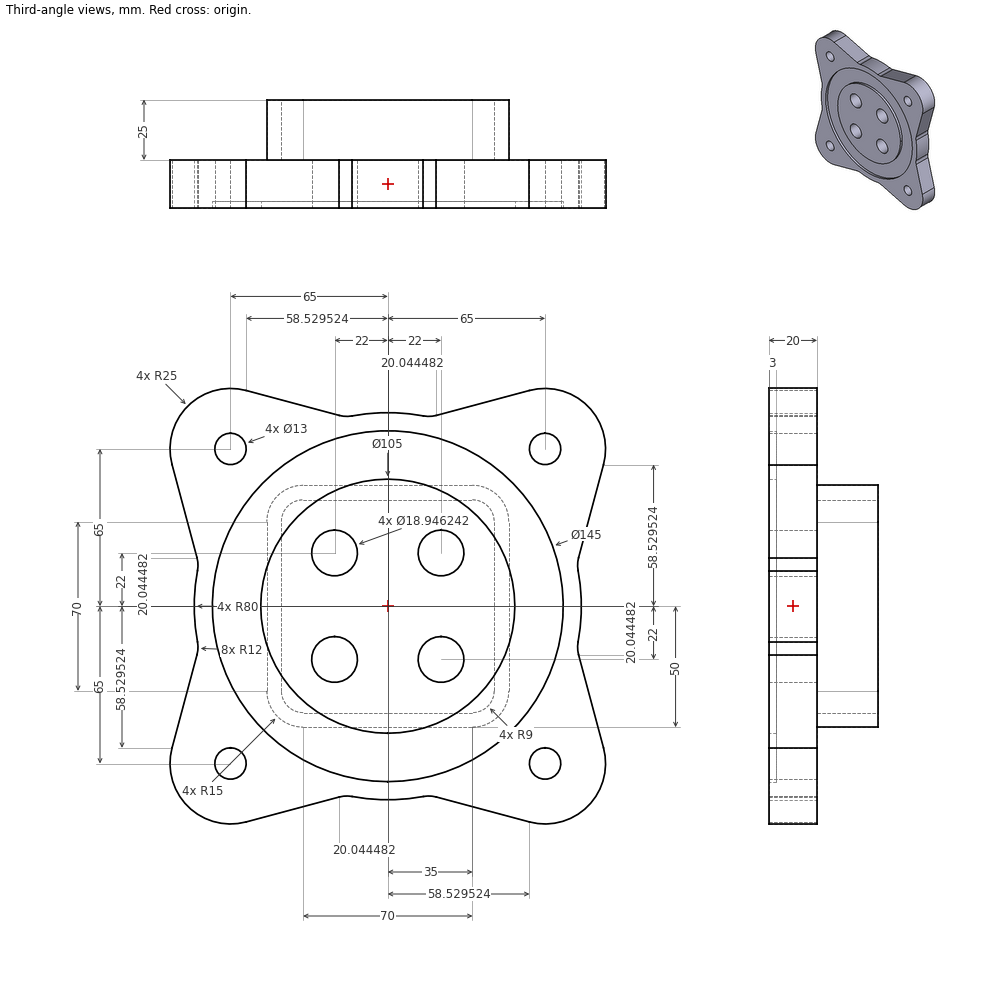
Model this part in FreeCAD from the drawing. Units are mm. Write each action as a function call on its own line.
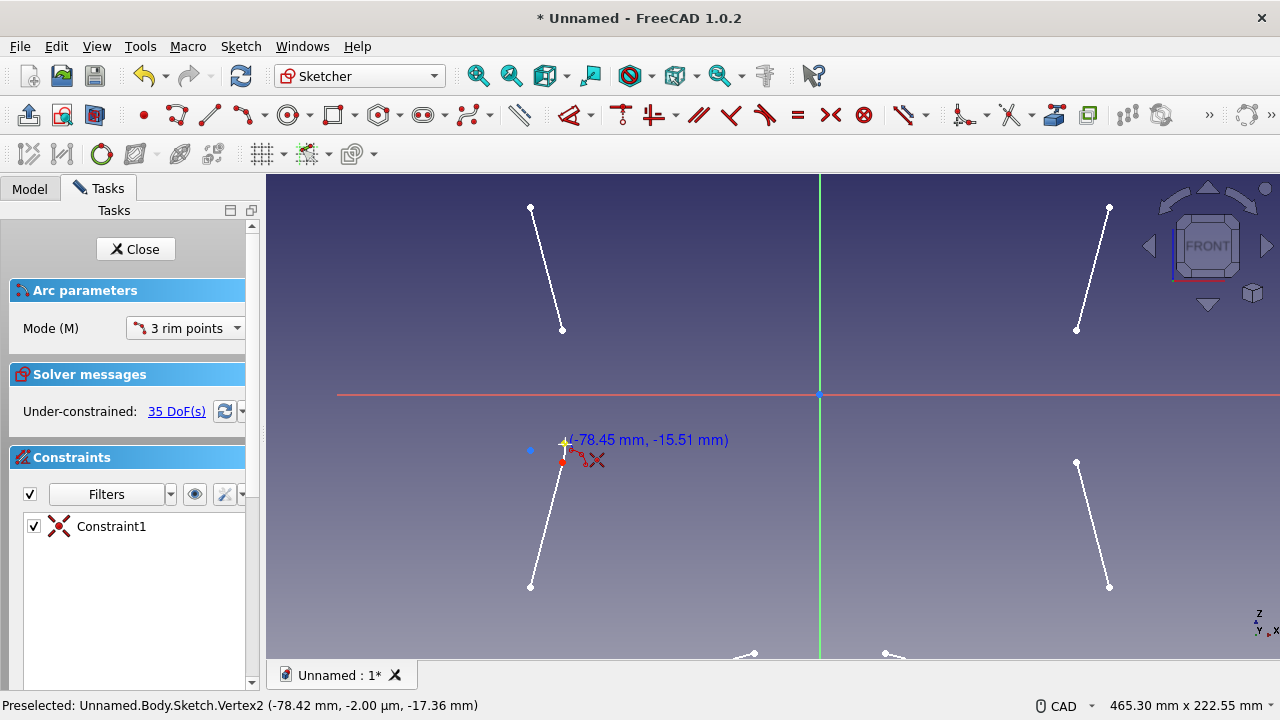
click(564, 444)
click(564, 347)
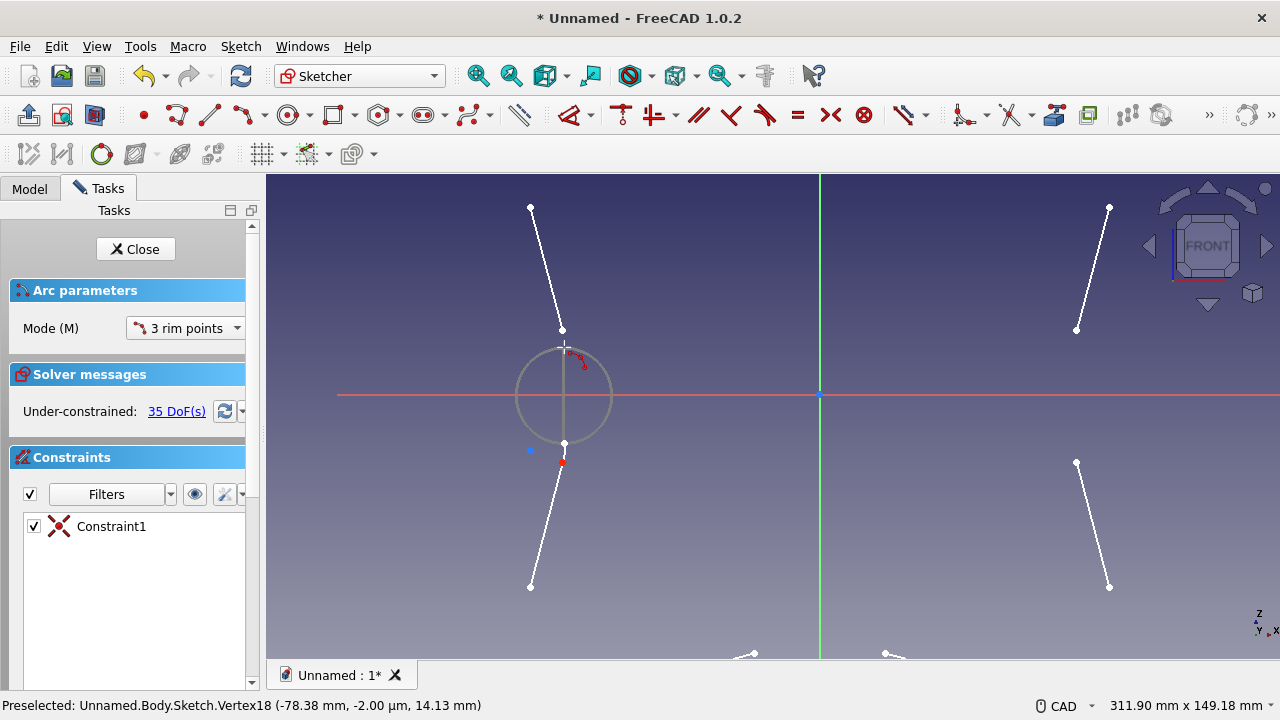
scroll(560, 385, up, 7)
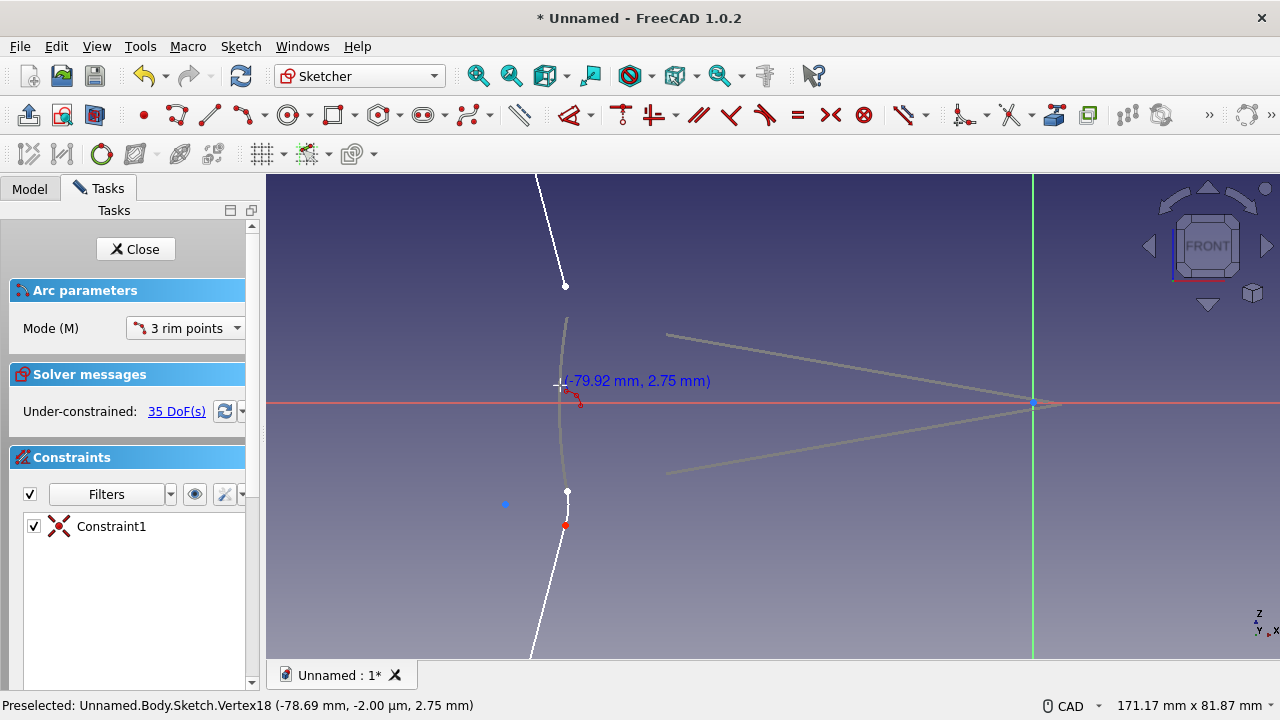
click(559, 385)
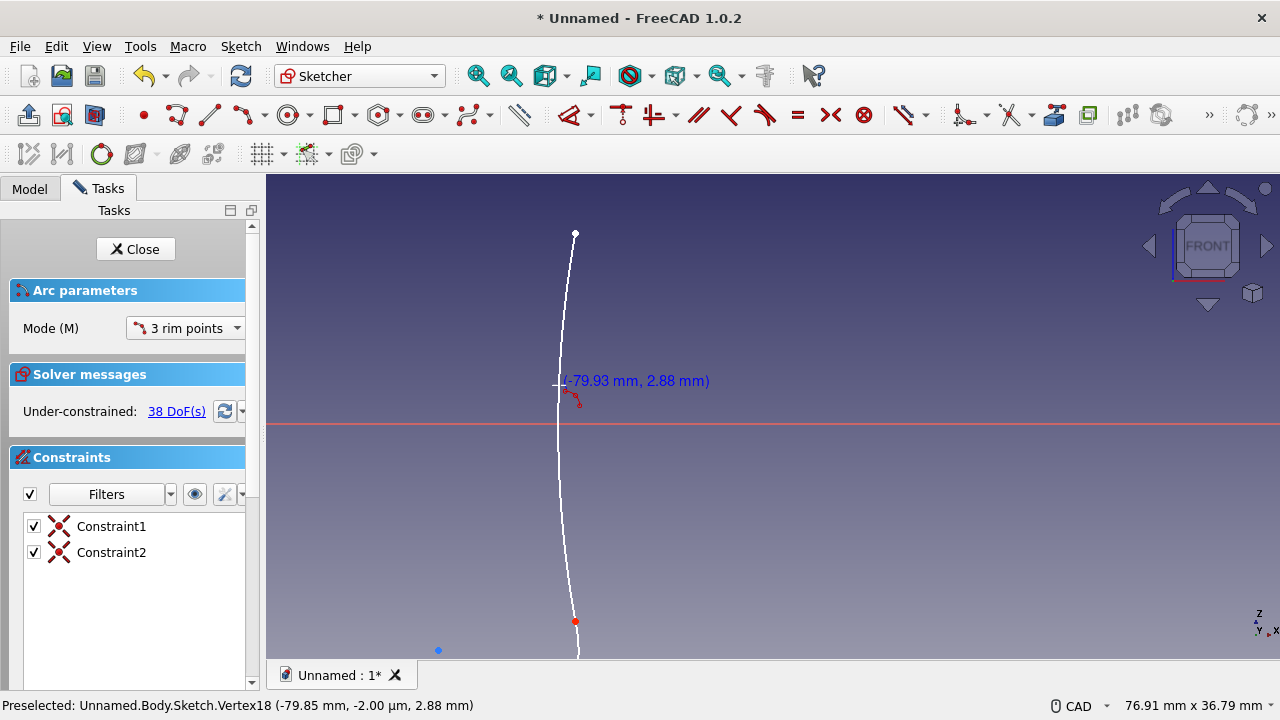
scroll(562, 415, down, 10)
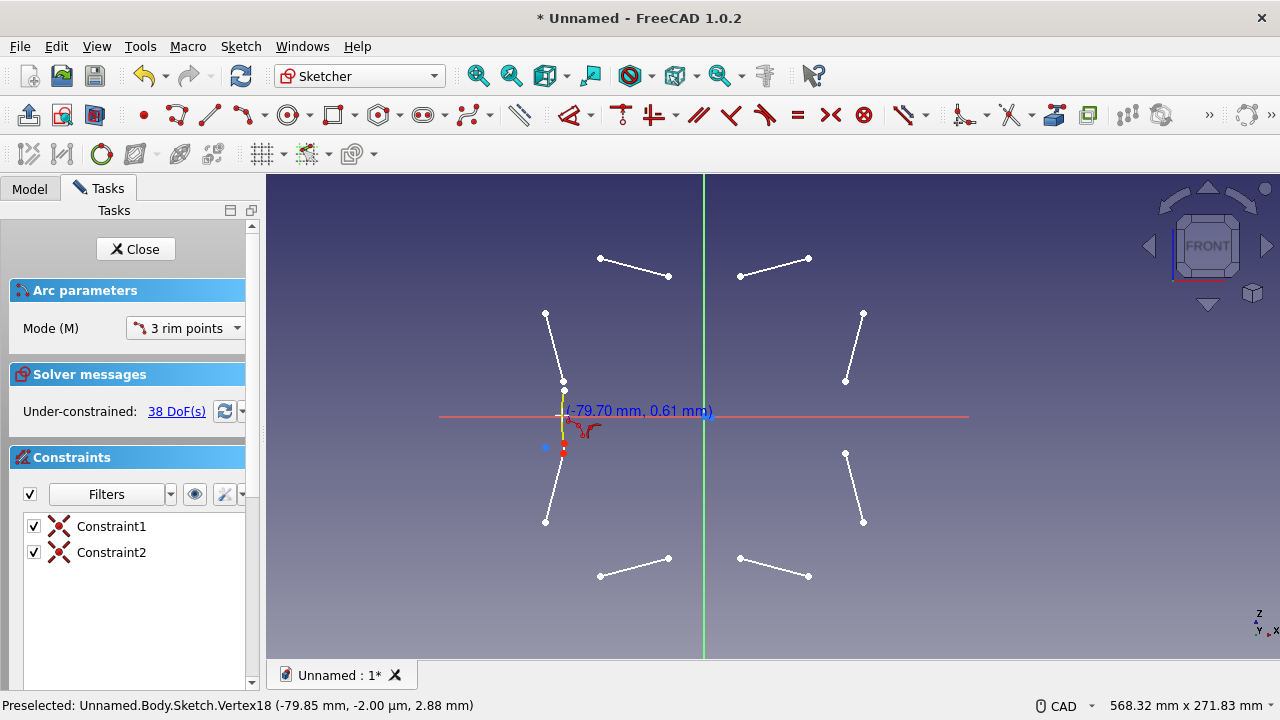
scroll(564, 390, up, 3)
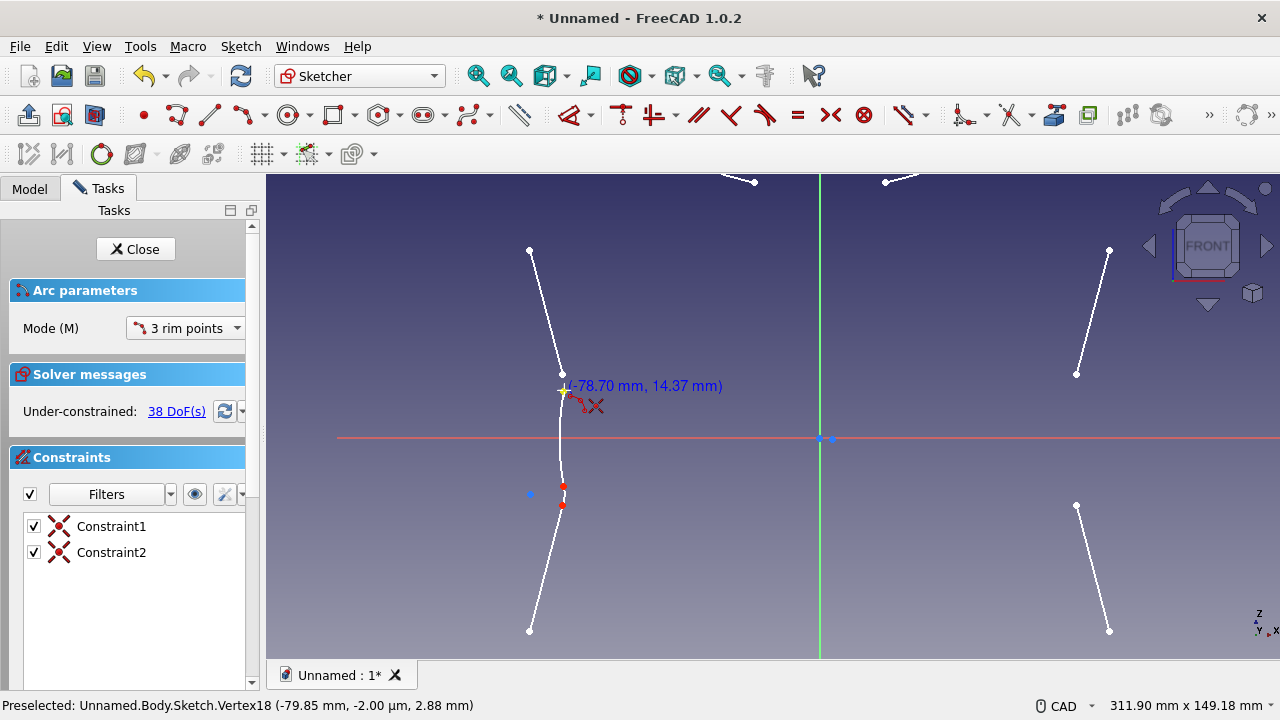
click(564, 391)
click(563, 374)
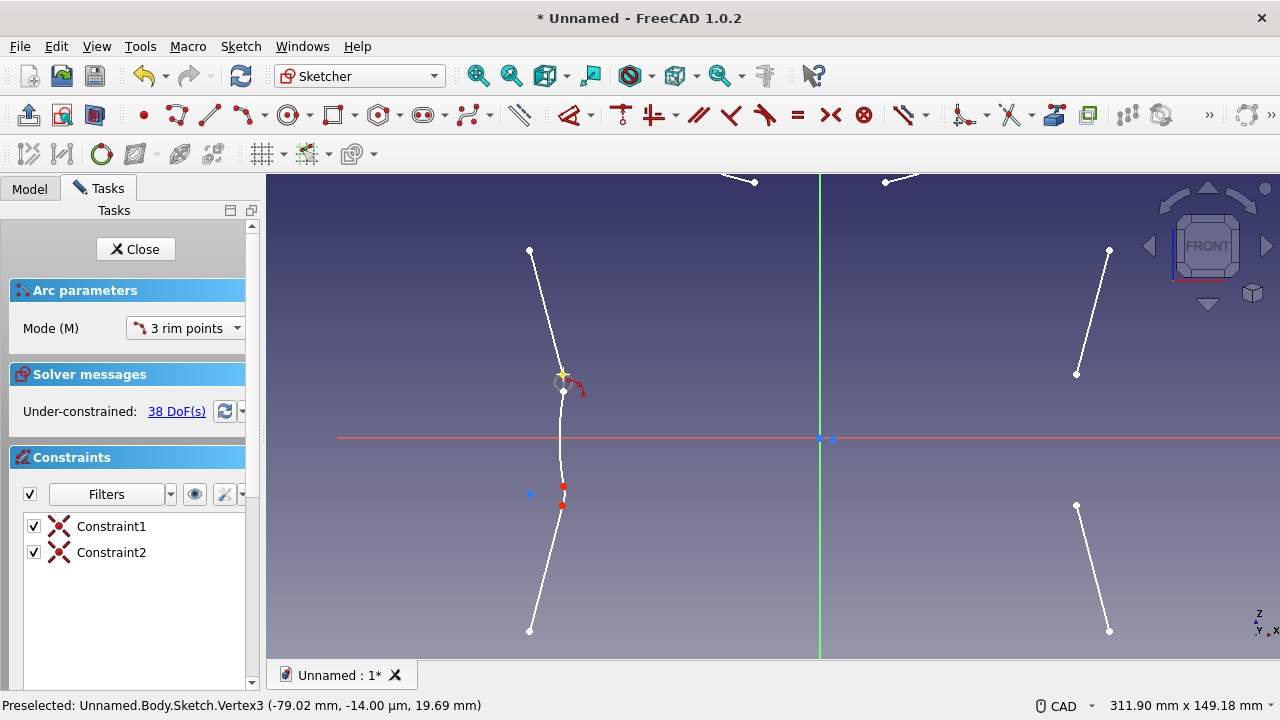
scroll(565, 382, up, 14)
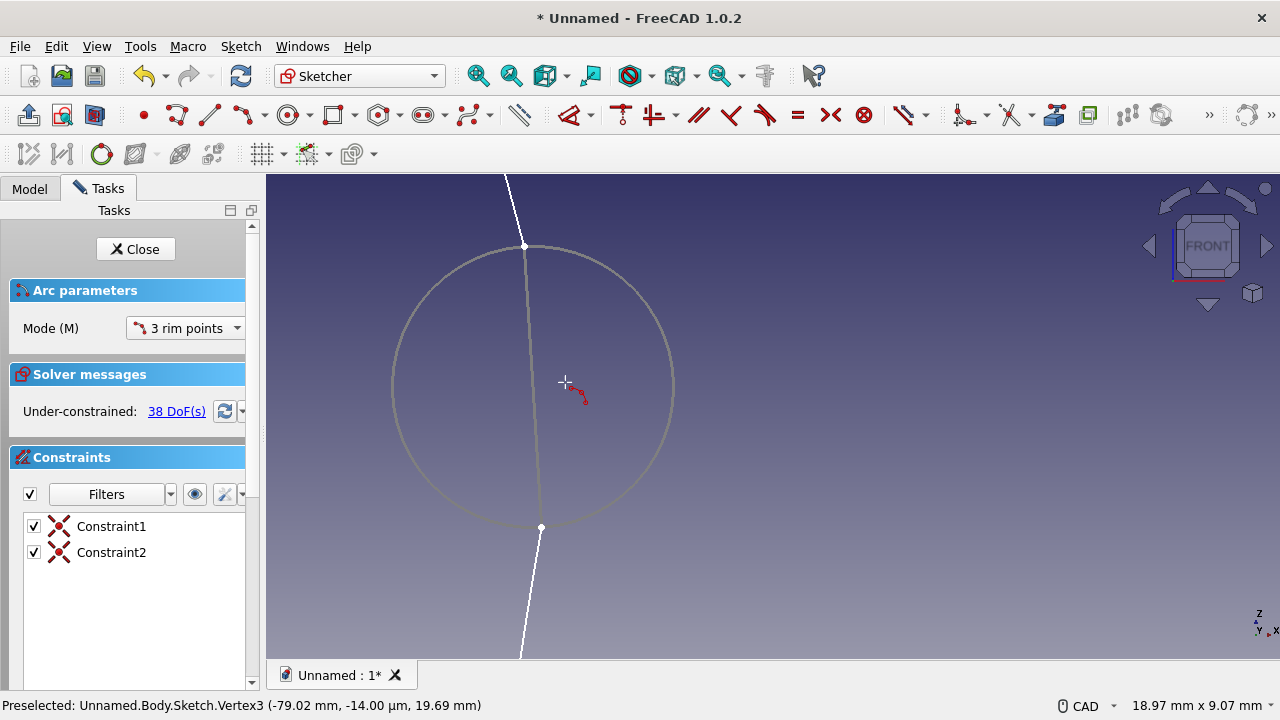
click(555, 369)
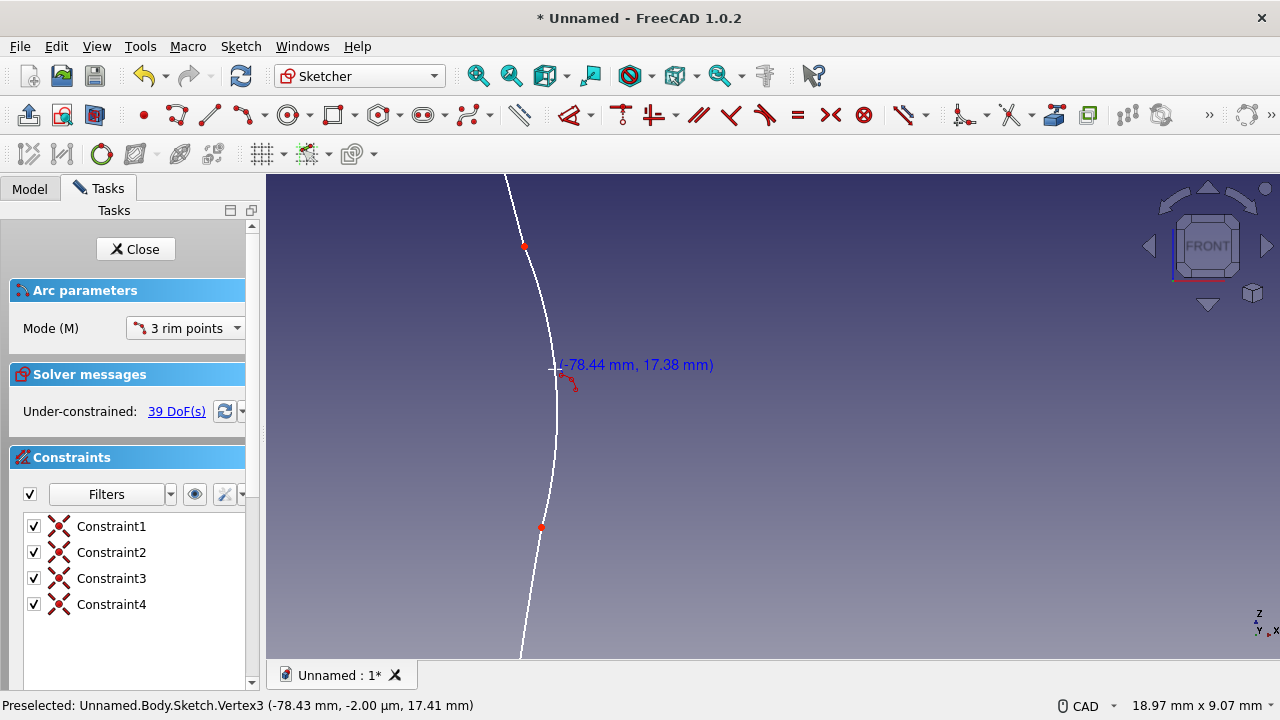
scroll(565, 386, down, 17)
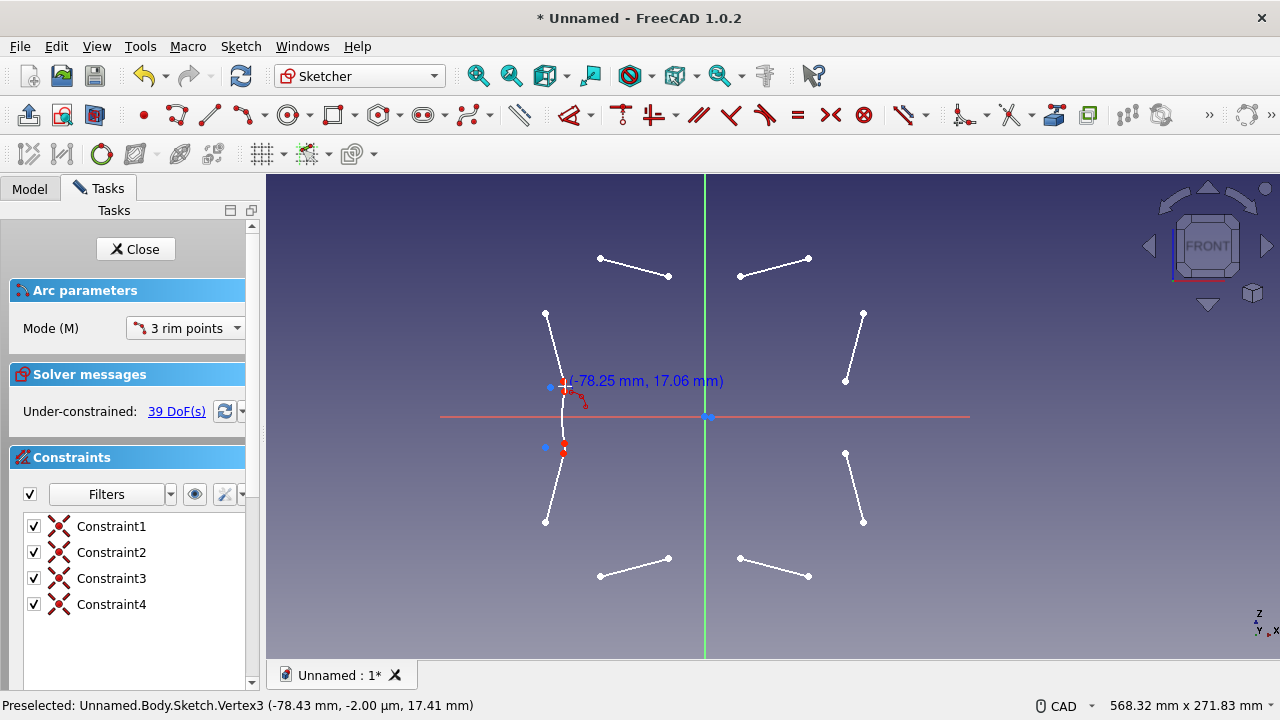
click(546, 314)
click(601, 259)
click(557, 269)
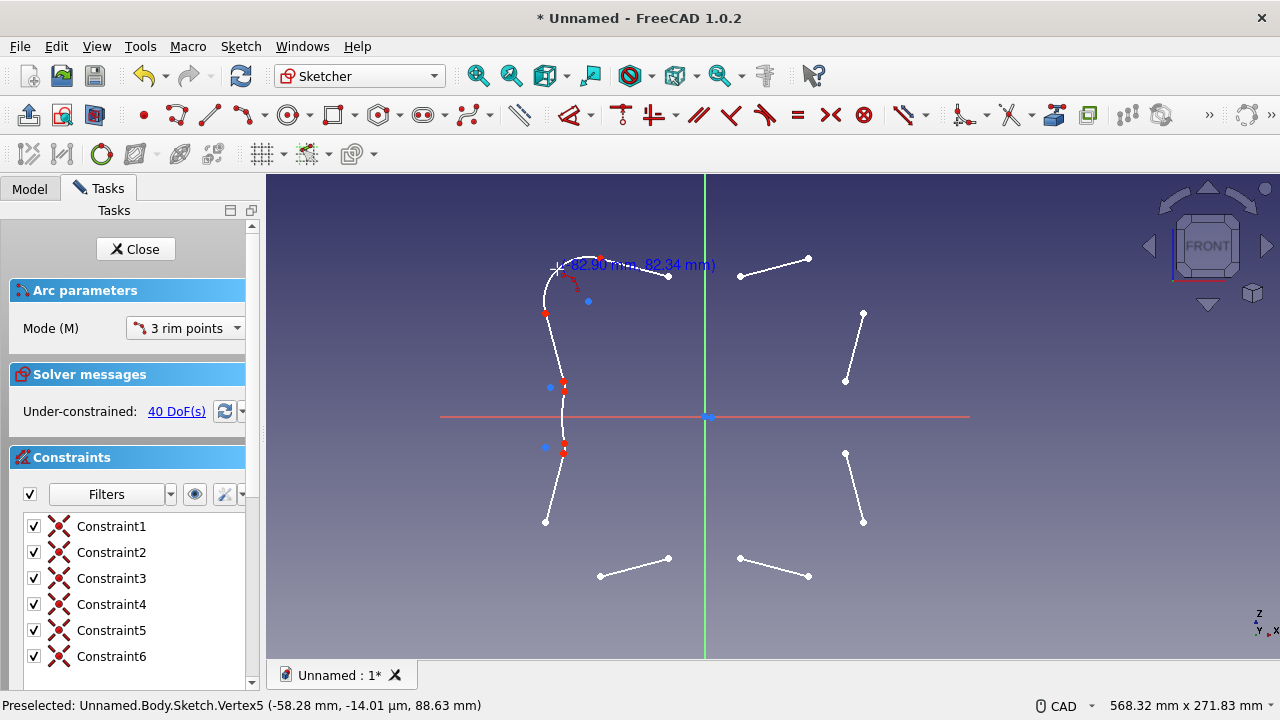
click(669, 277)